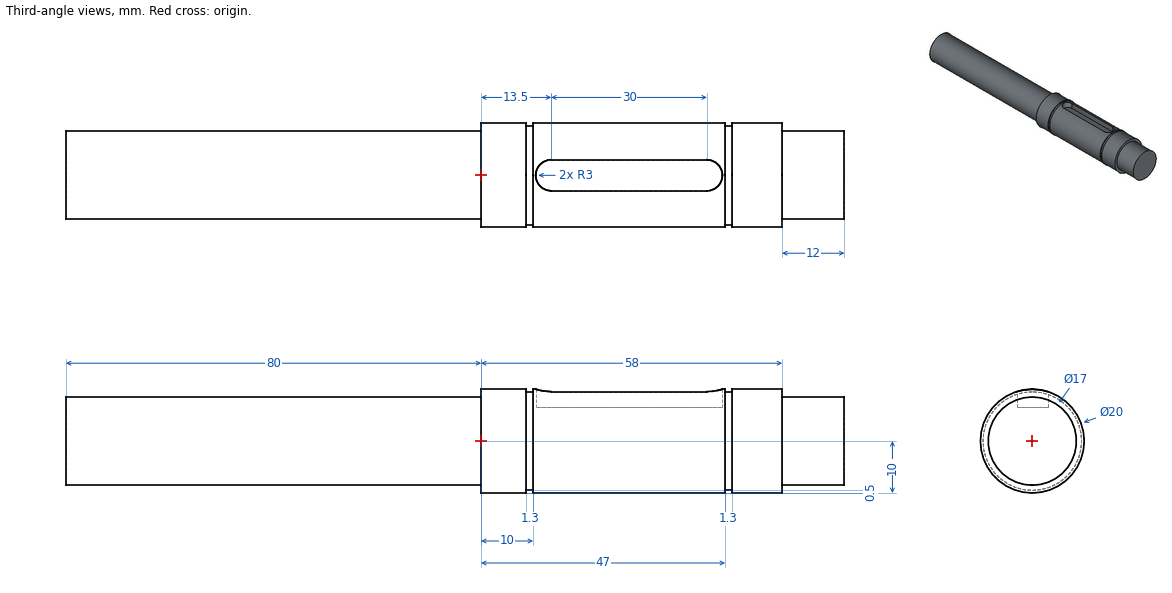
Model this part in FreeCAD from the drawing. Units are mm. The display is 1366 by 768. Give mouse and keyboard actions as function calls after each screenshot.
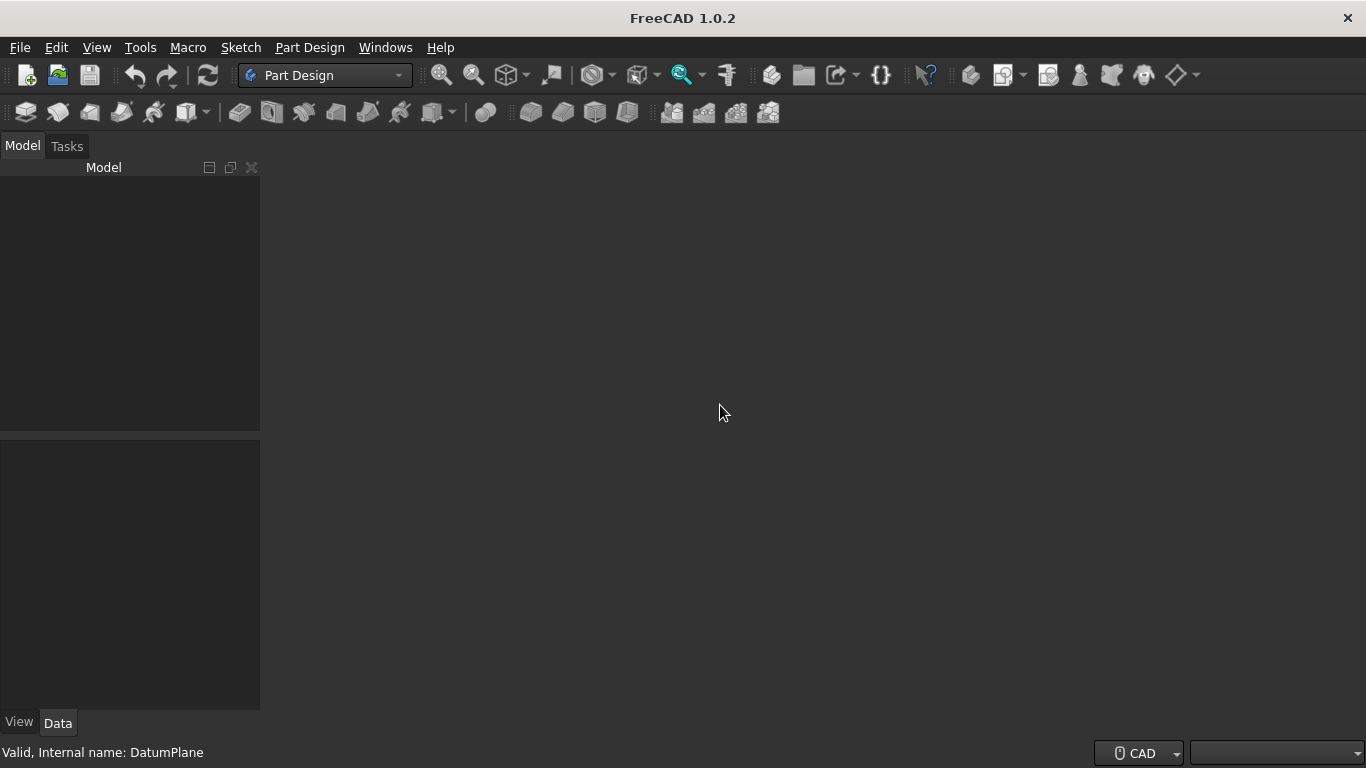
key(ctrl+n)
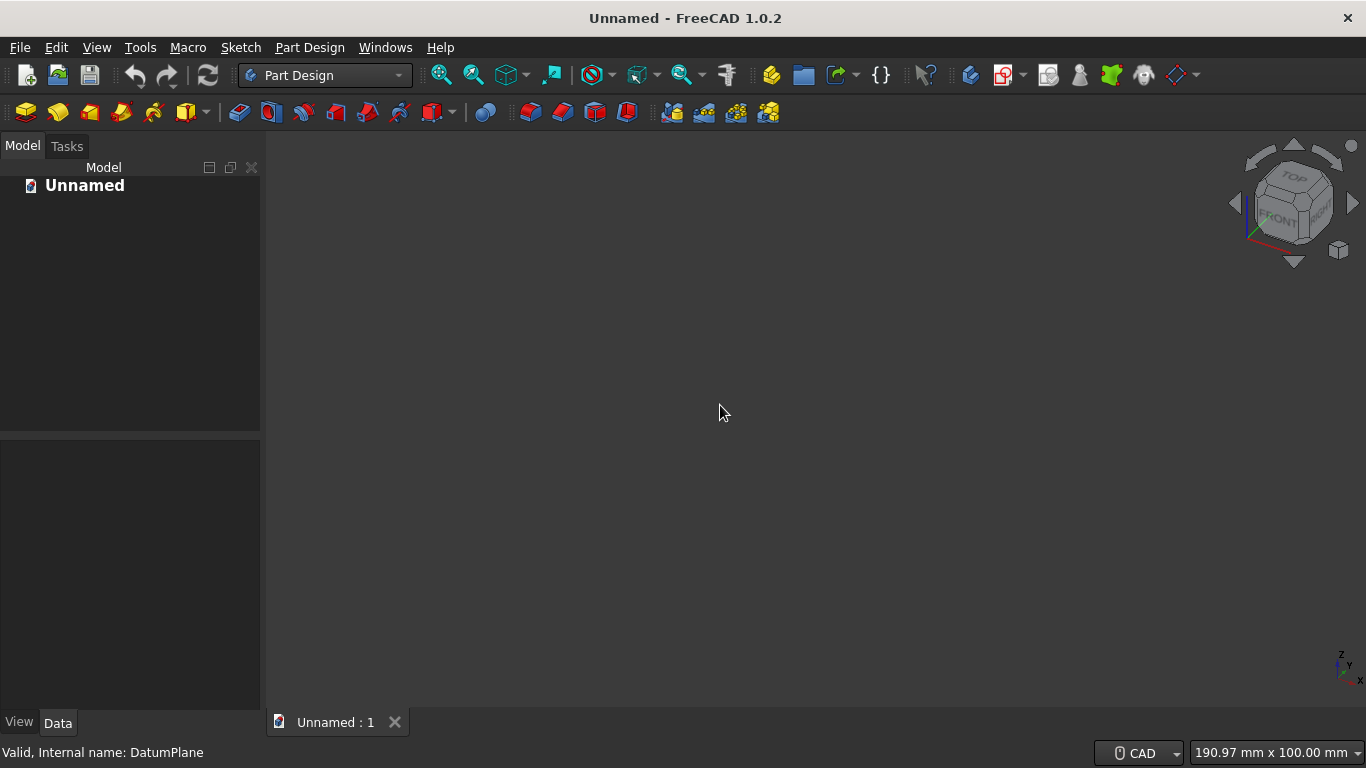
click(1004, 76)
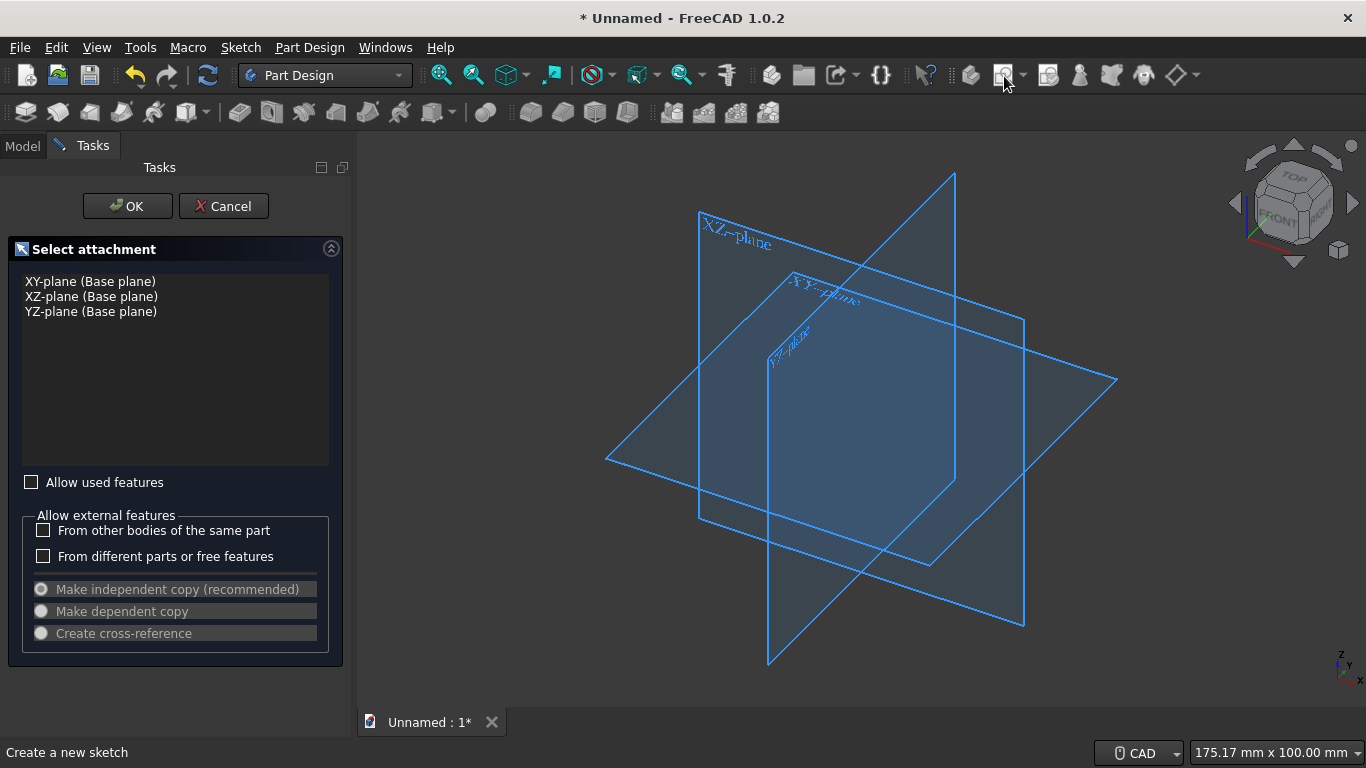
click(82, 312)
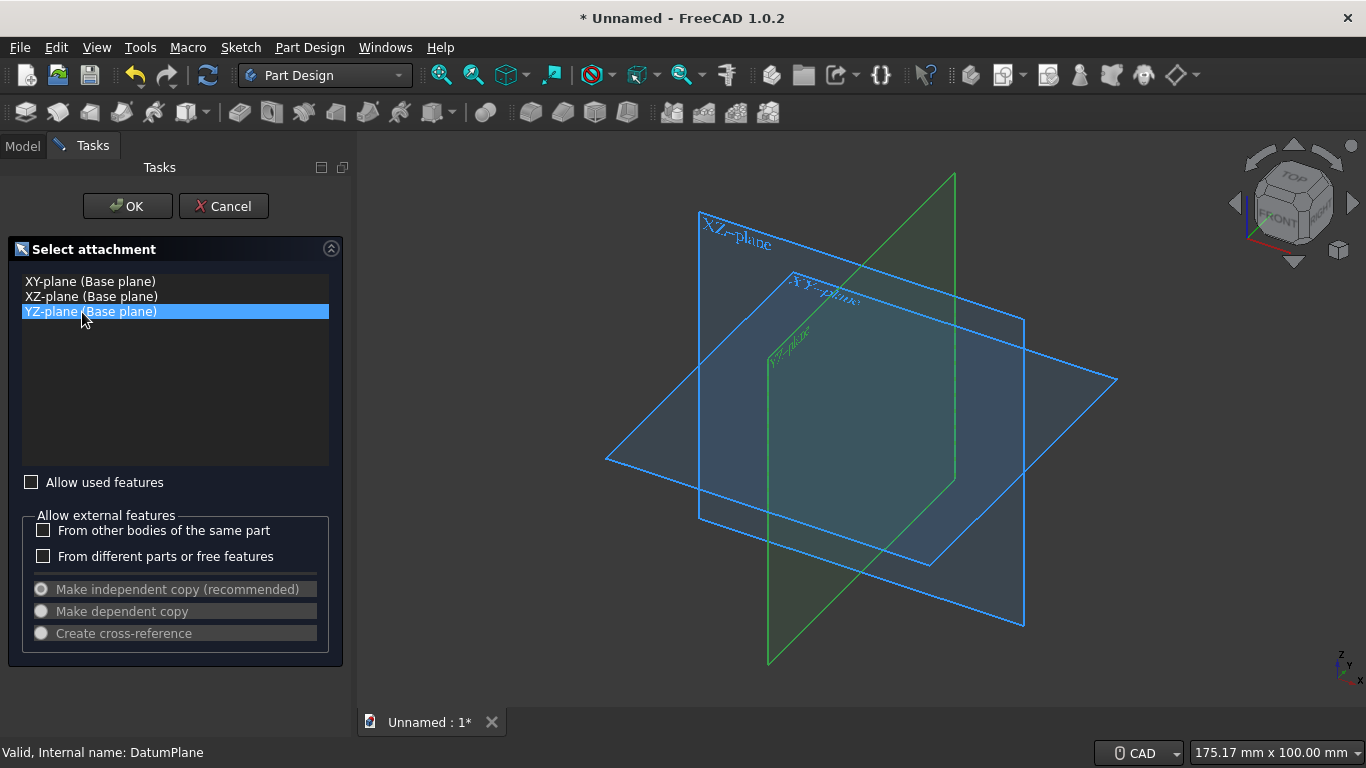
click(128, 206)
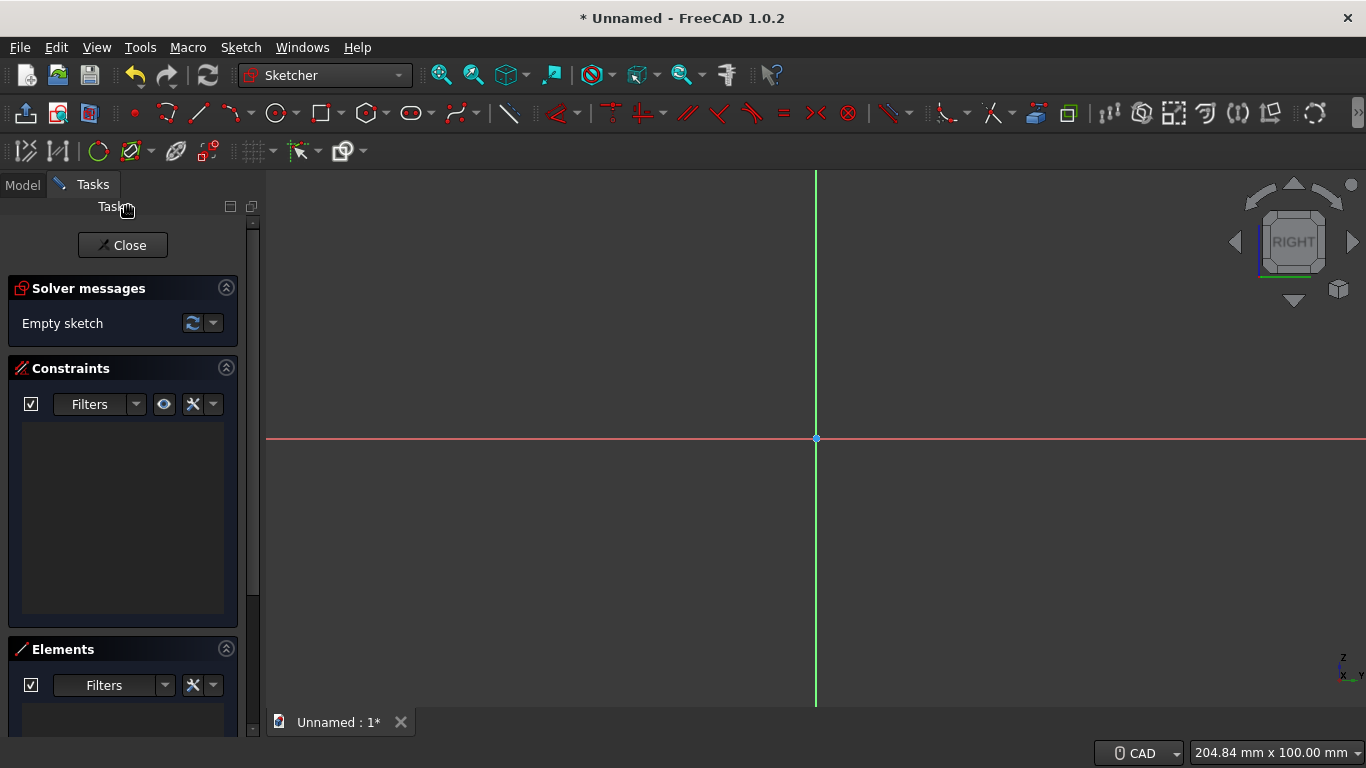
scroll(846, 438, up, 6)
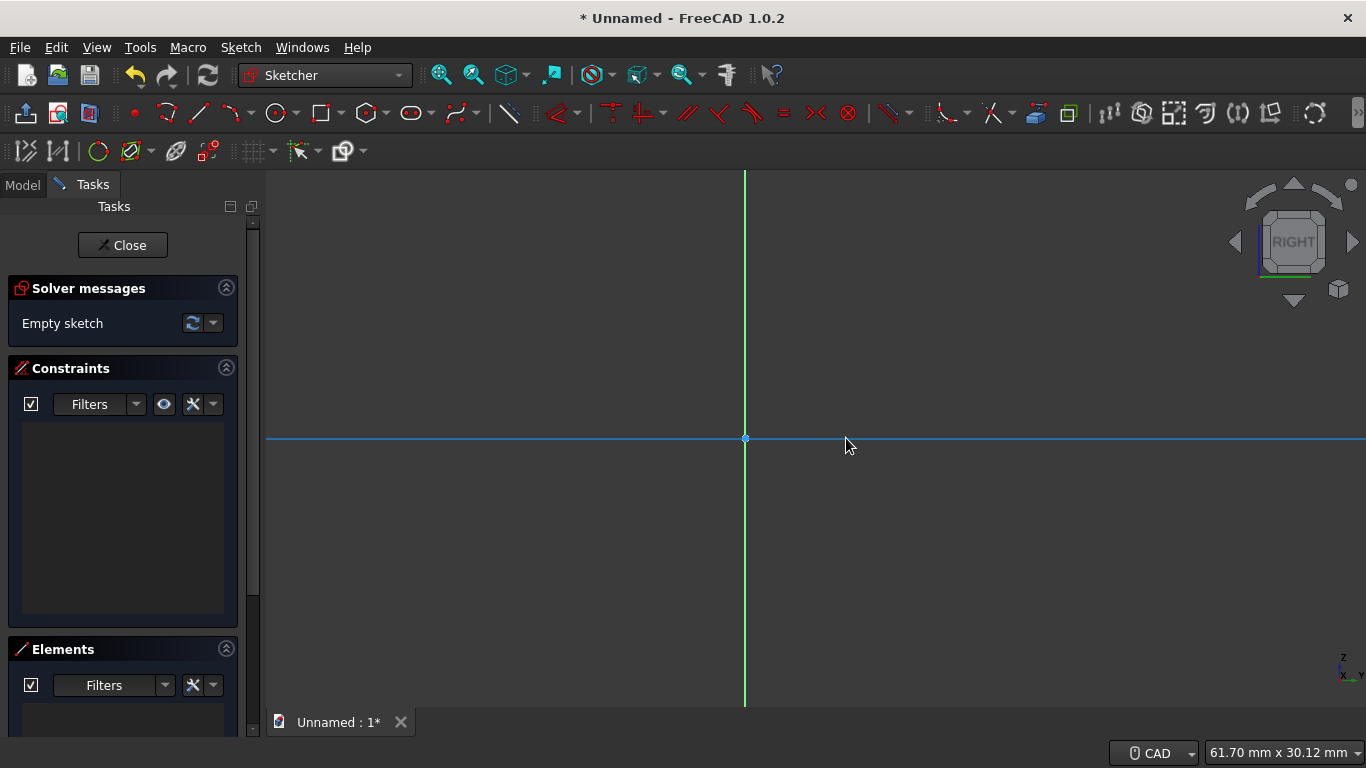
click(276, 114)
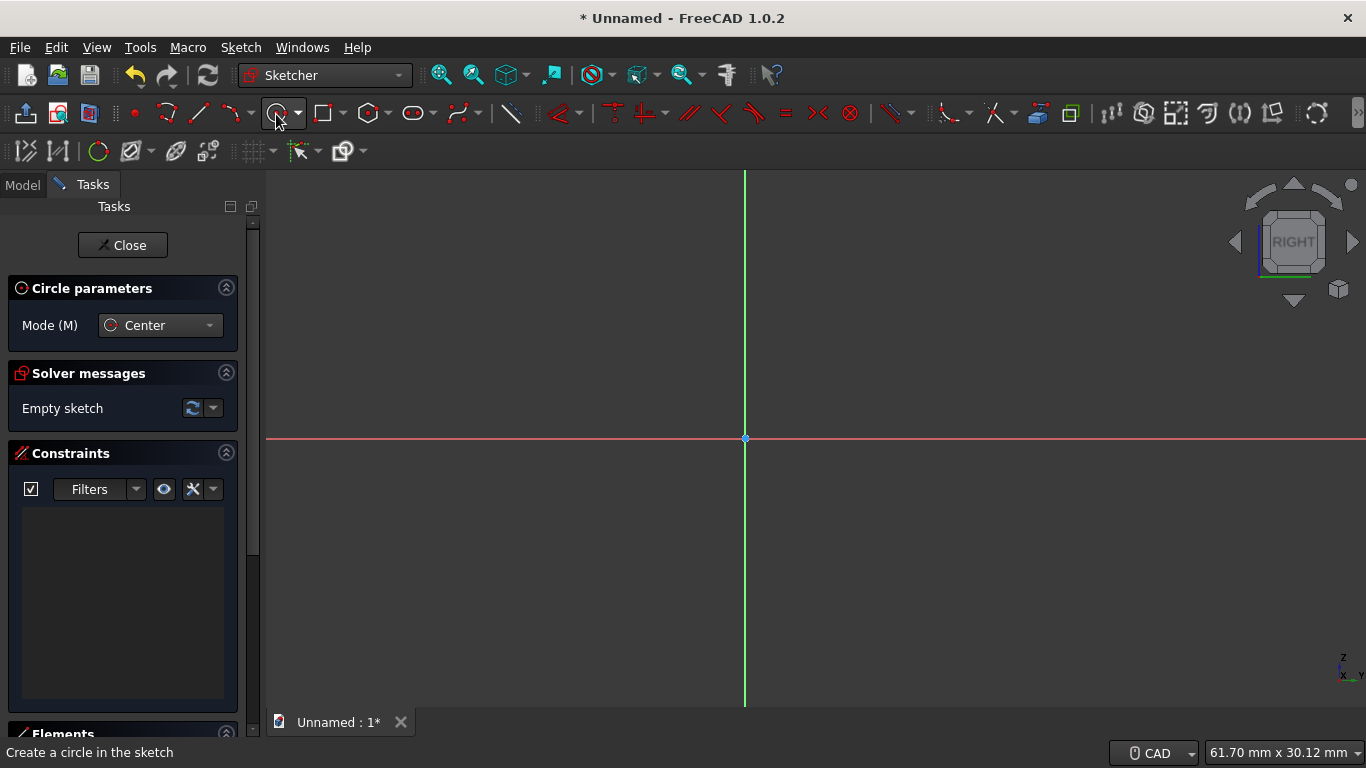
click(745, 438)
click(871, 312)
key(Escape)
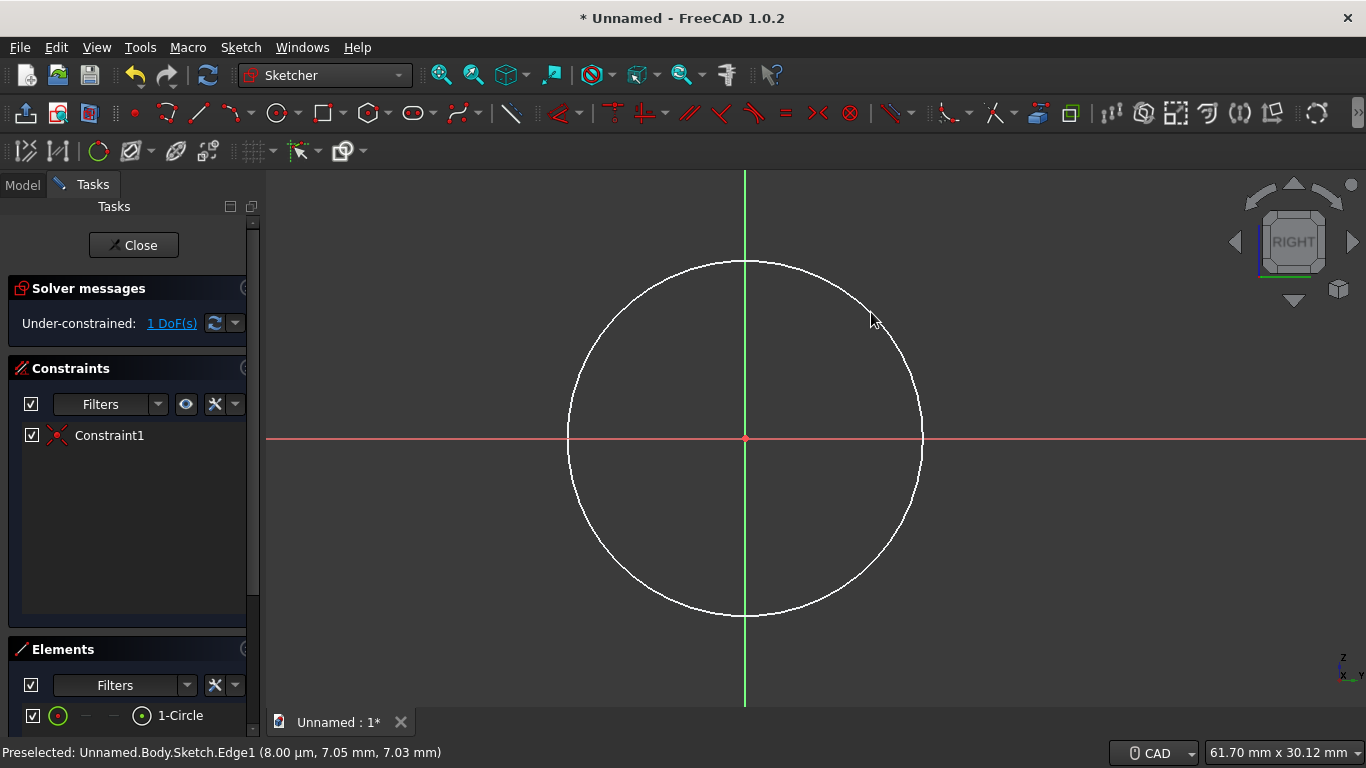
click(558, 114)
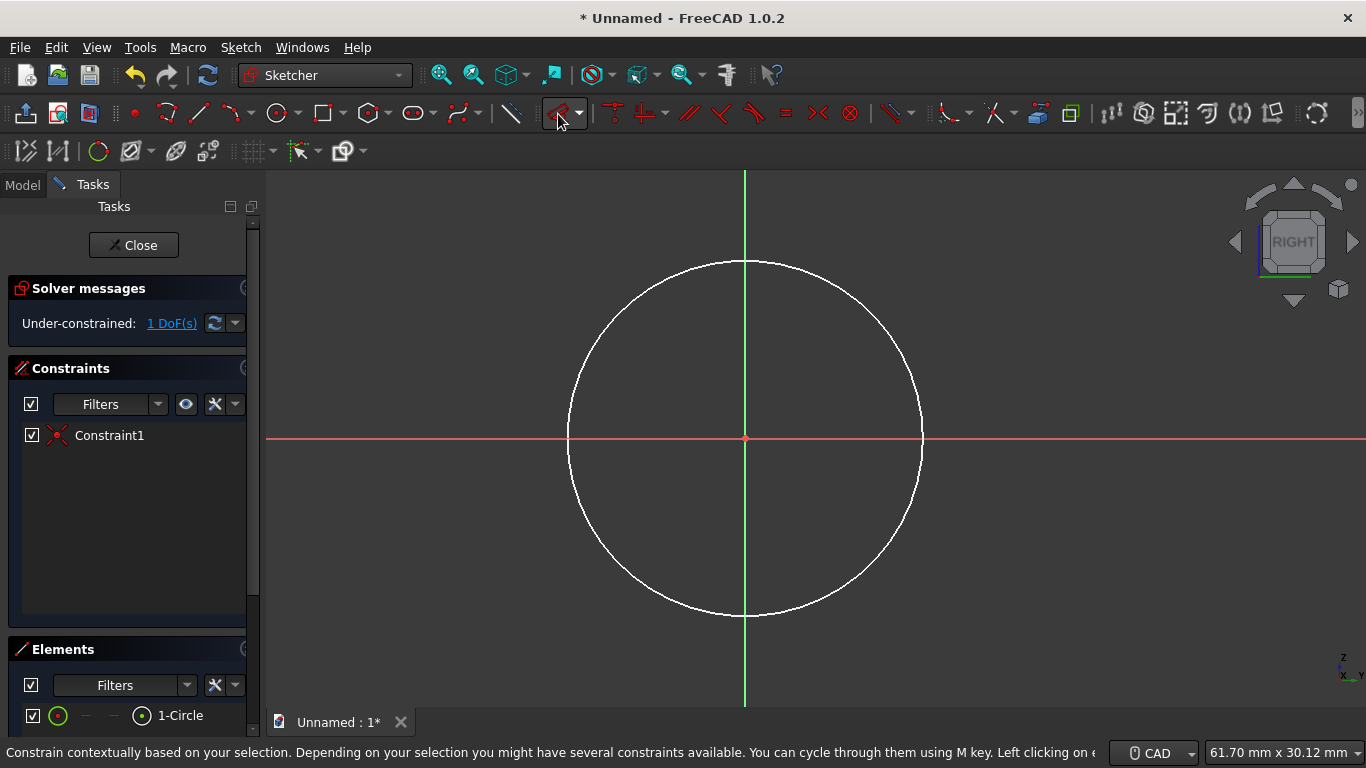
click(870, 312)
click(892, 289)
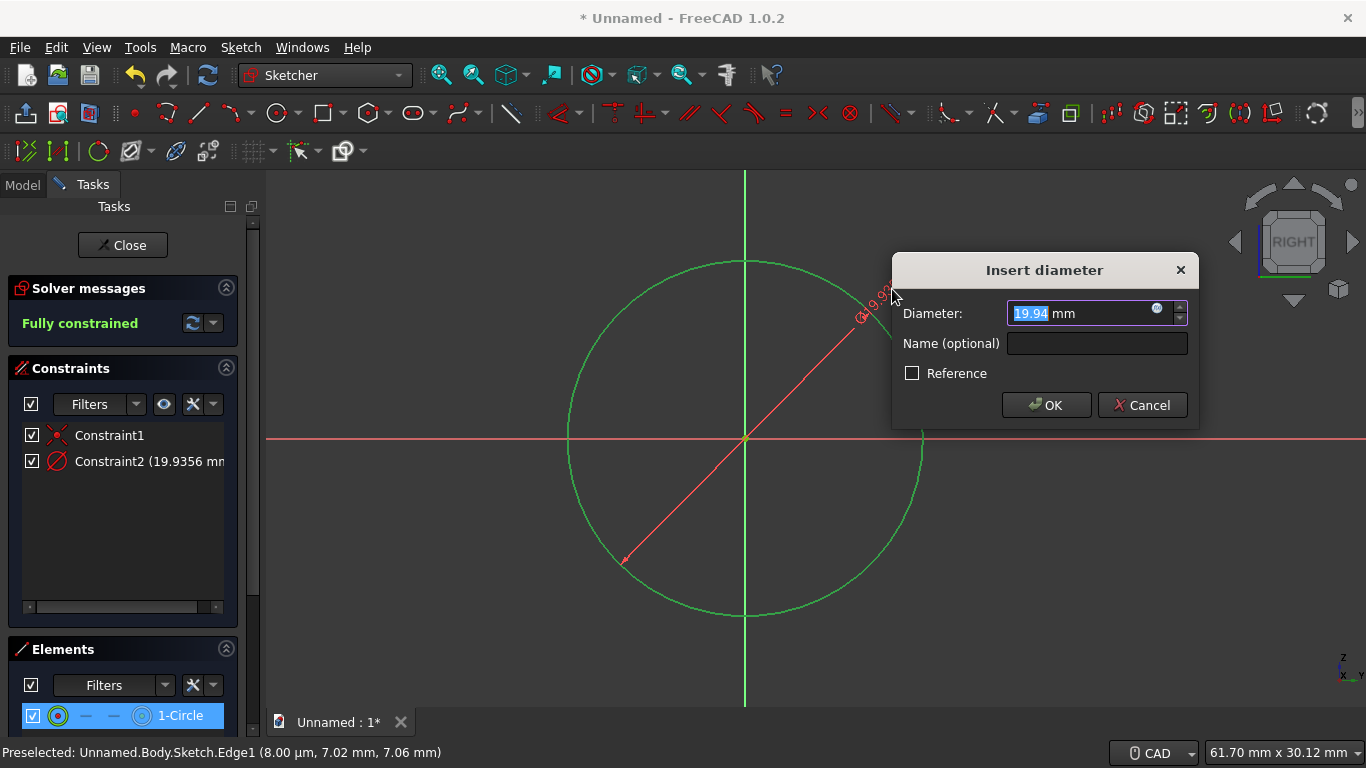
text(20)
key(Return)
key(Escape)